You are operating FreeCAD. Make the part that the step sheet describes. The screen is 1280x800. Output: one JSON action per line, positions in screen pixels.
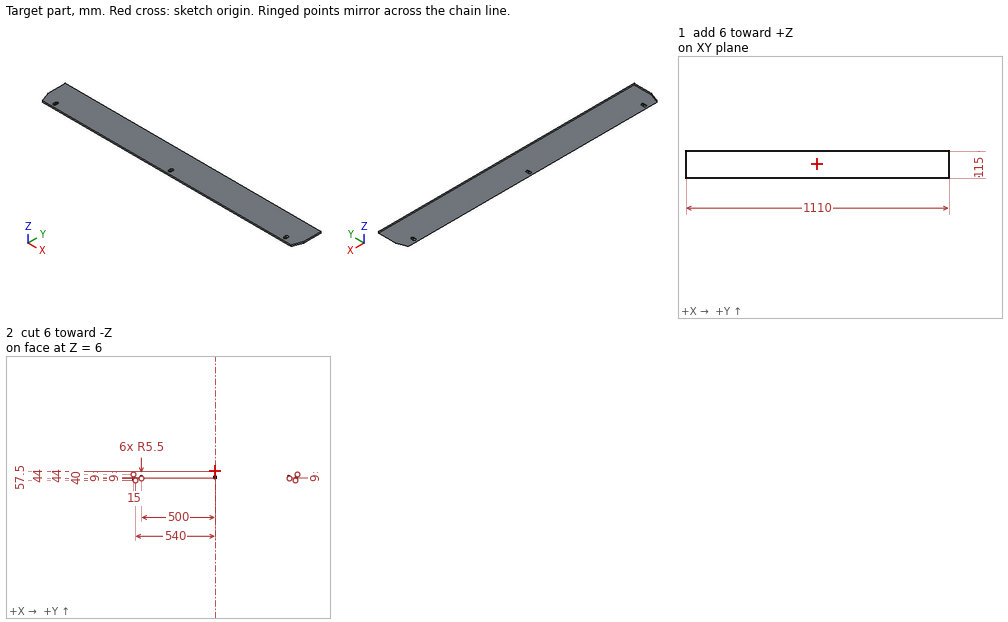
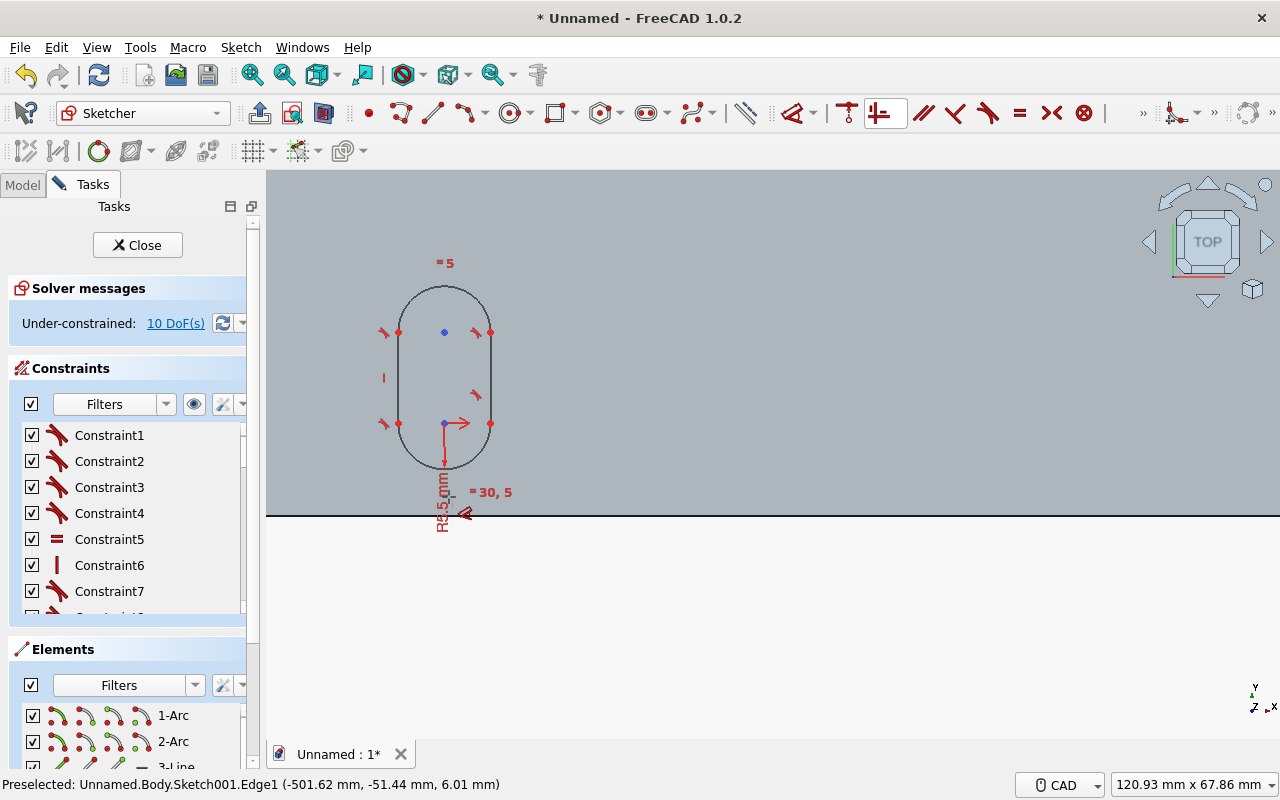
{"action": "left_click", "coordinate": [398, 396]}
{"action": "left_click", "coordinate": [364, 378]}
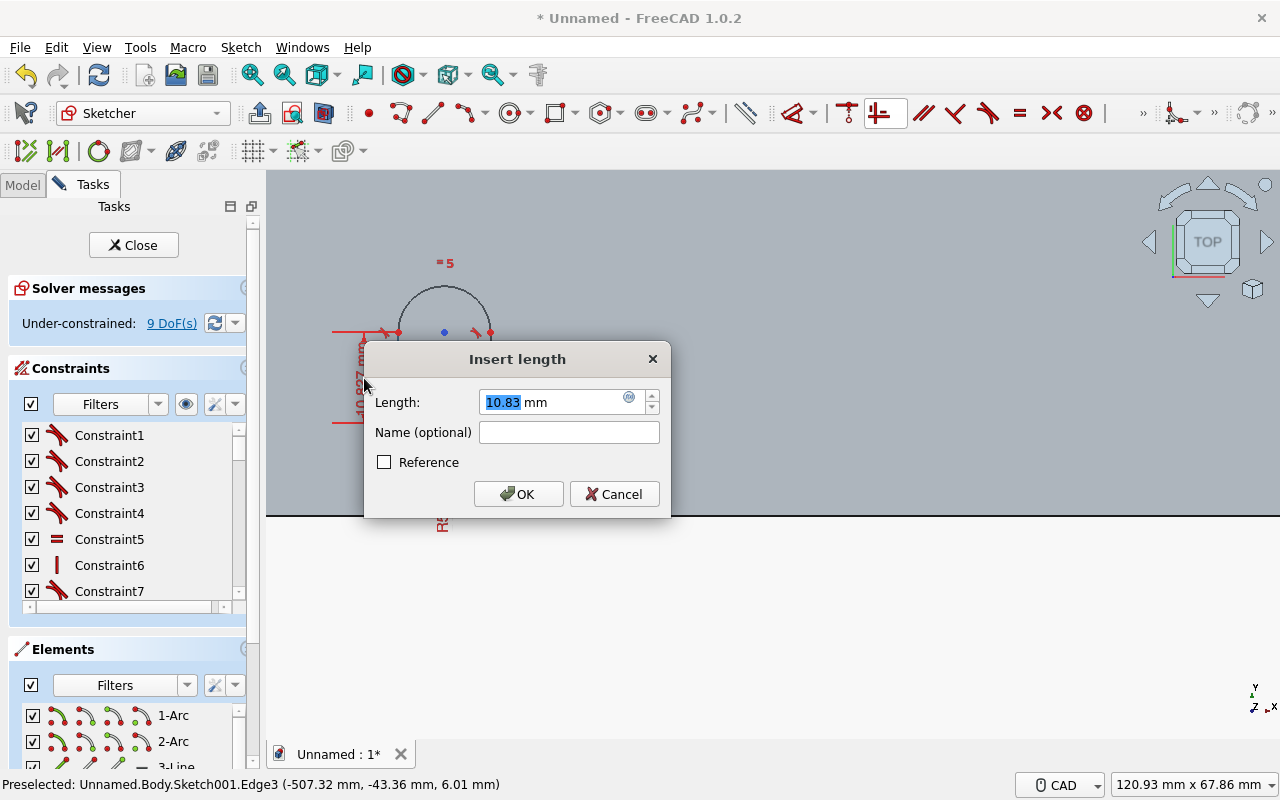
{"action": "type", "text": "9"}
{"action": "key", "text": "Return"}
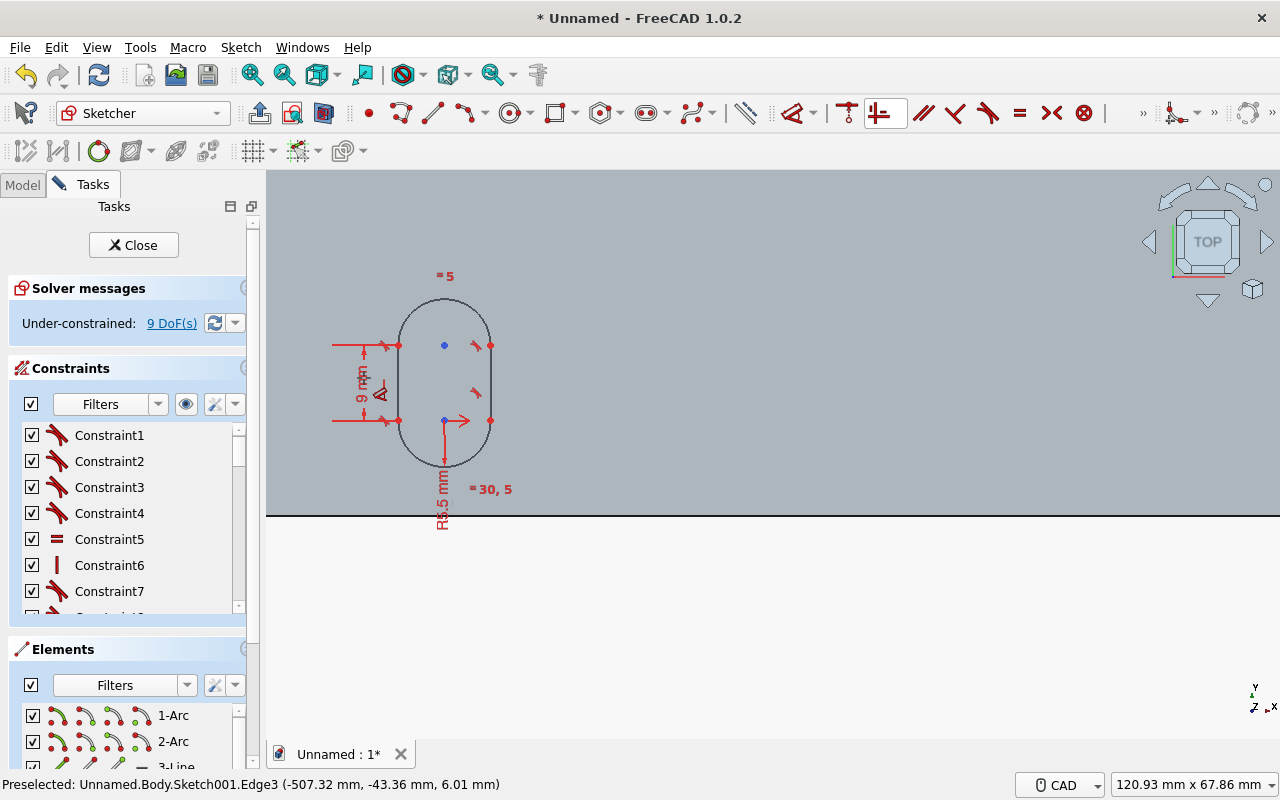
{"action": "scroll", "coordinate": [449, 466], "scroll_direction": "down", "scroll_amount": 14}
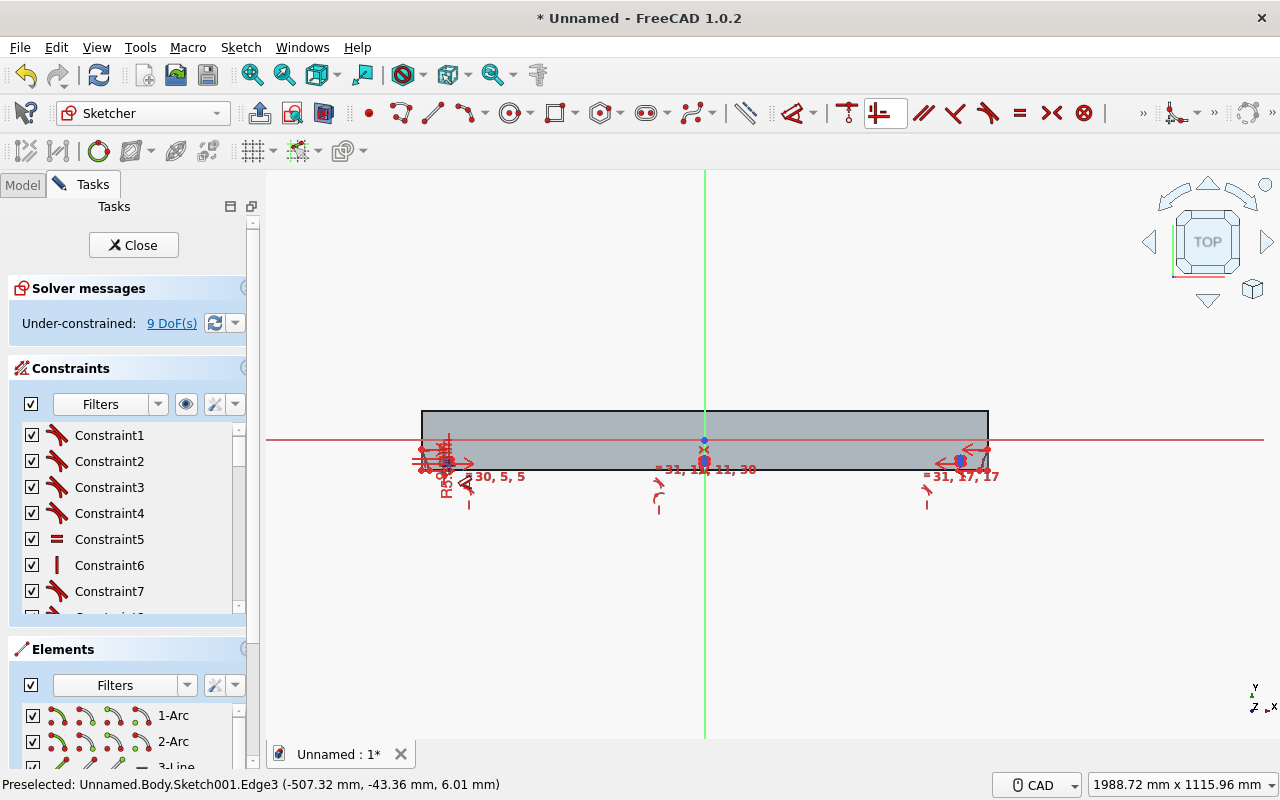
{"action": "scroll", "coordinate": [702, 462], "scroll_direction": "up", "scroll_amount": 13}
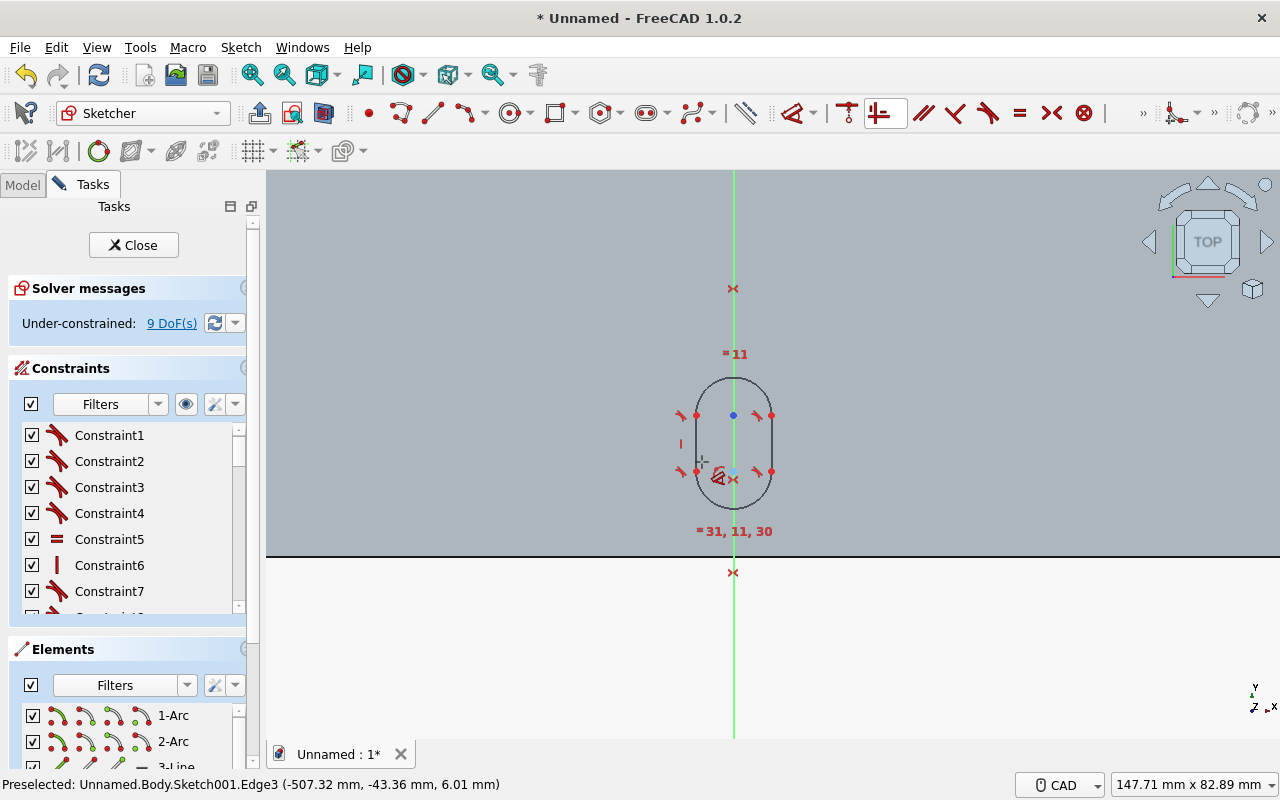
{"action": "left_click", "coordinate": [696, 454]}
{"action": "left_click", "coordinate": [662, 443]}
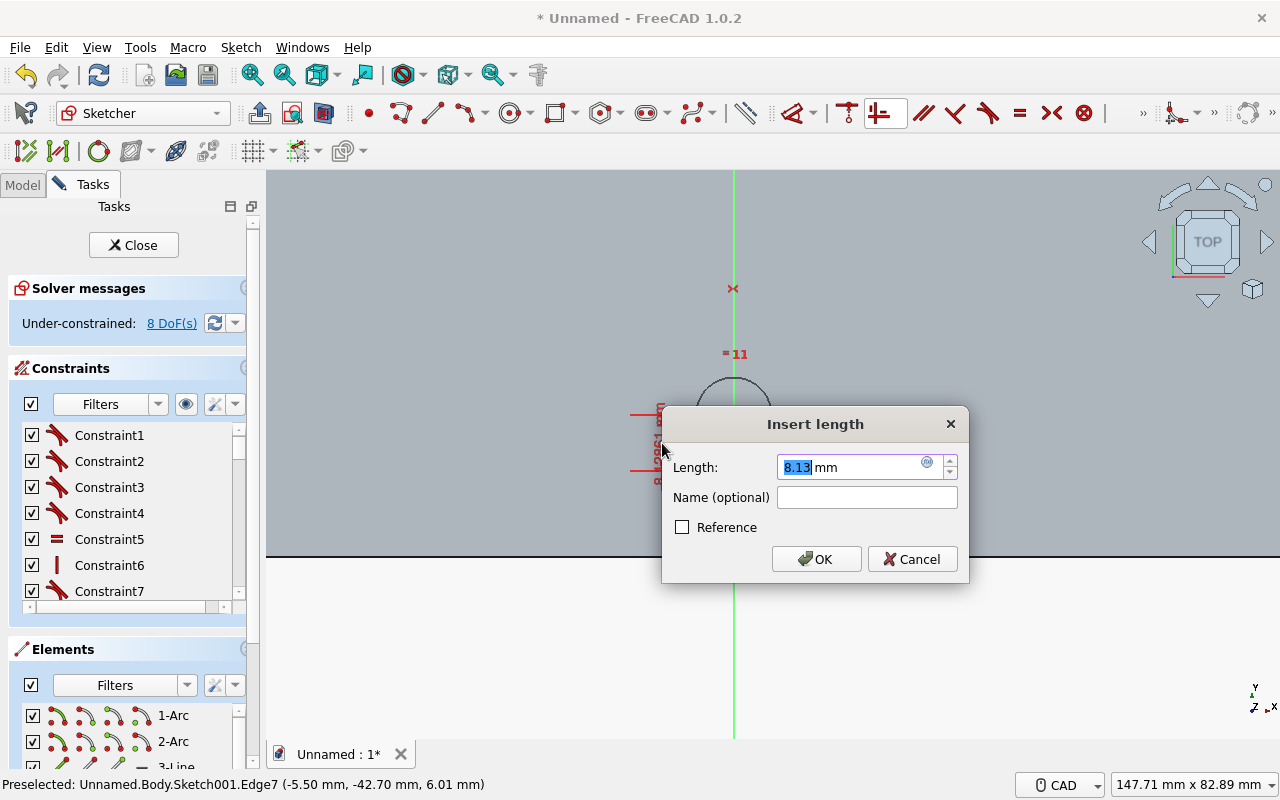
{"action": "type", "text": "9"}
{"action": "key", "text": "Return"}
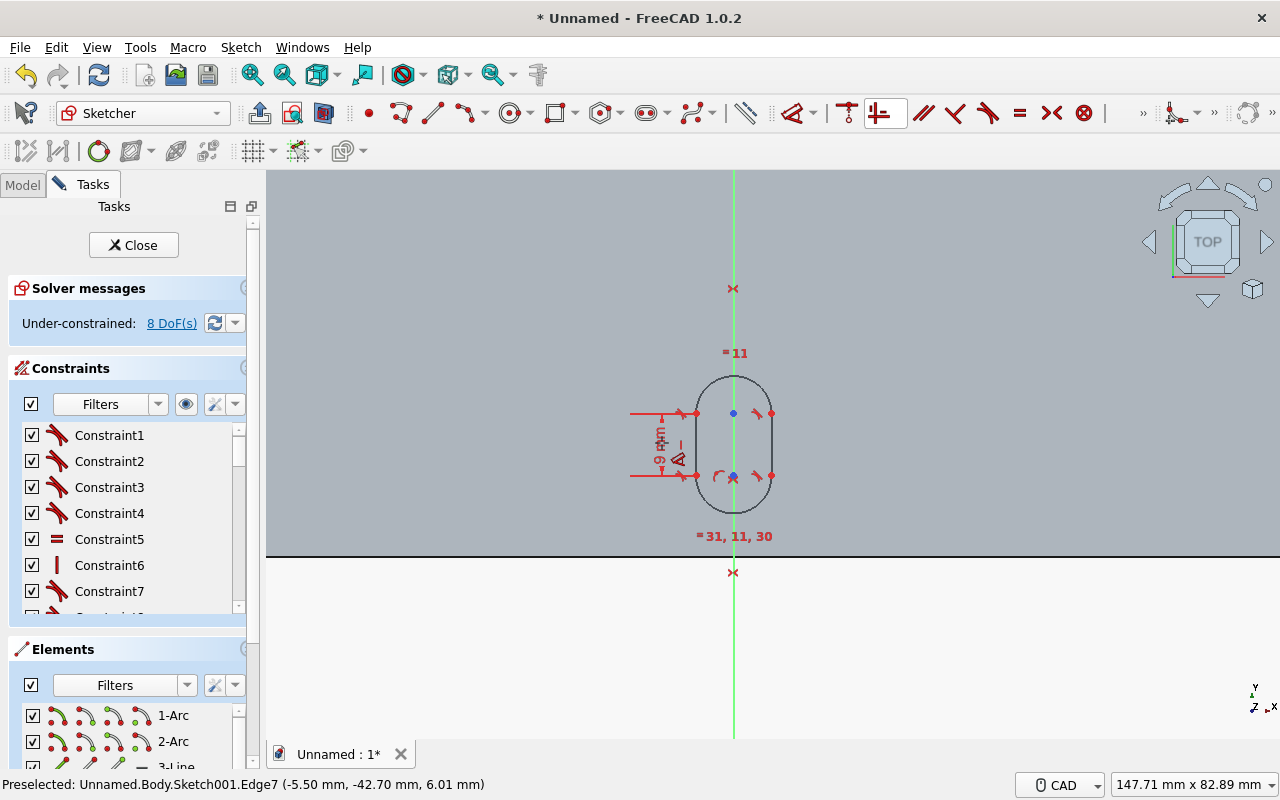
{"action": "scroll", "coordinate": [702, 462], "scroll_direction": "down", "scroll_amount": 13}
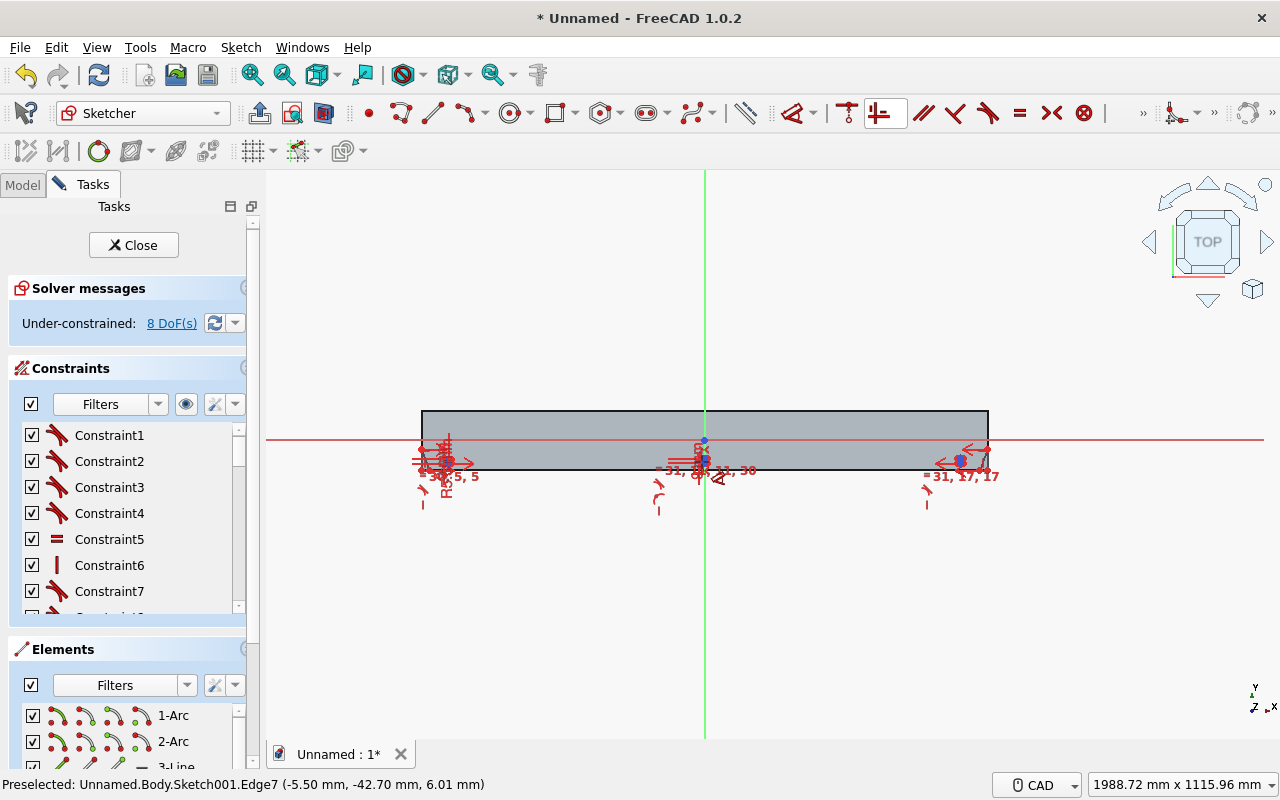
{"action": "scroll", "coordinate": [958, 462], "scroll_direction": "up", "scroll_amount": 11}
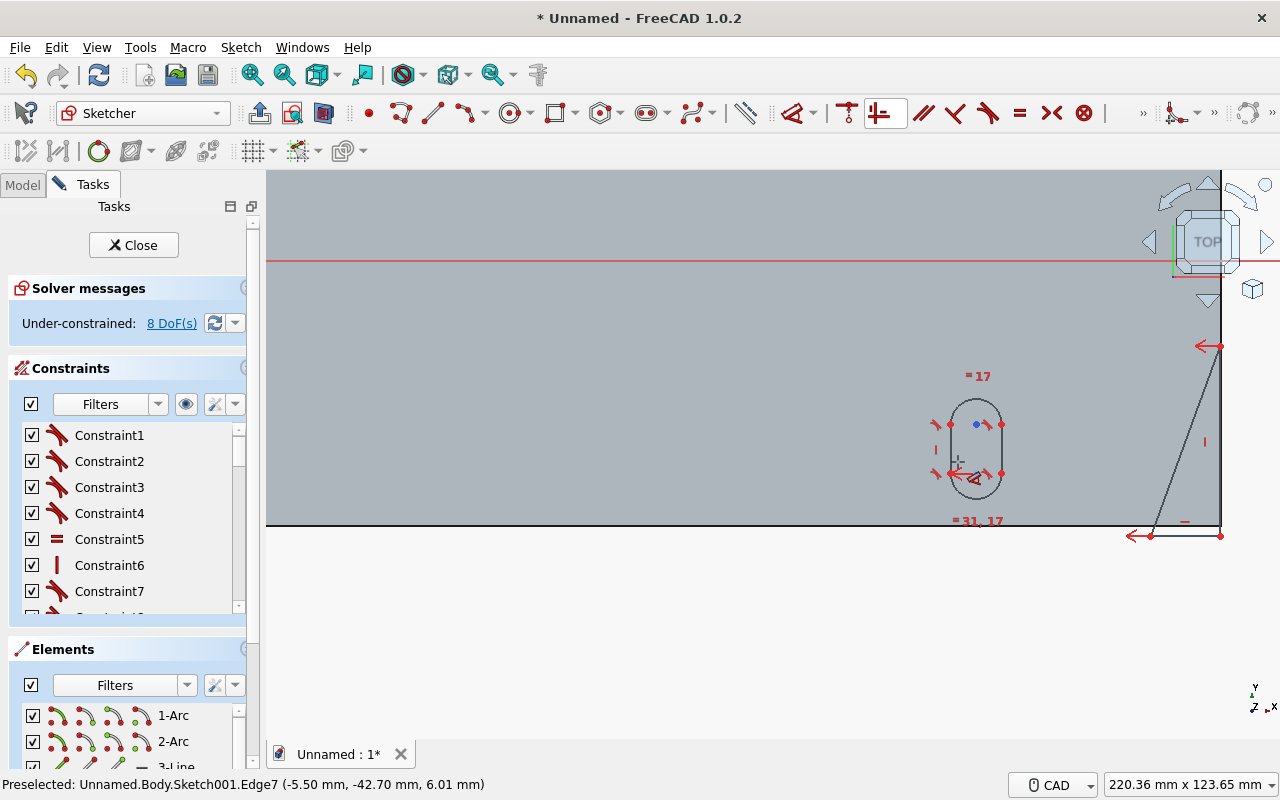
{"action": "left_click", "coordinate": [951, 459]}
{"action": "left_click", "coordinate": [985, 449]}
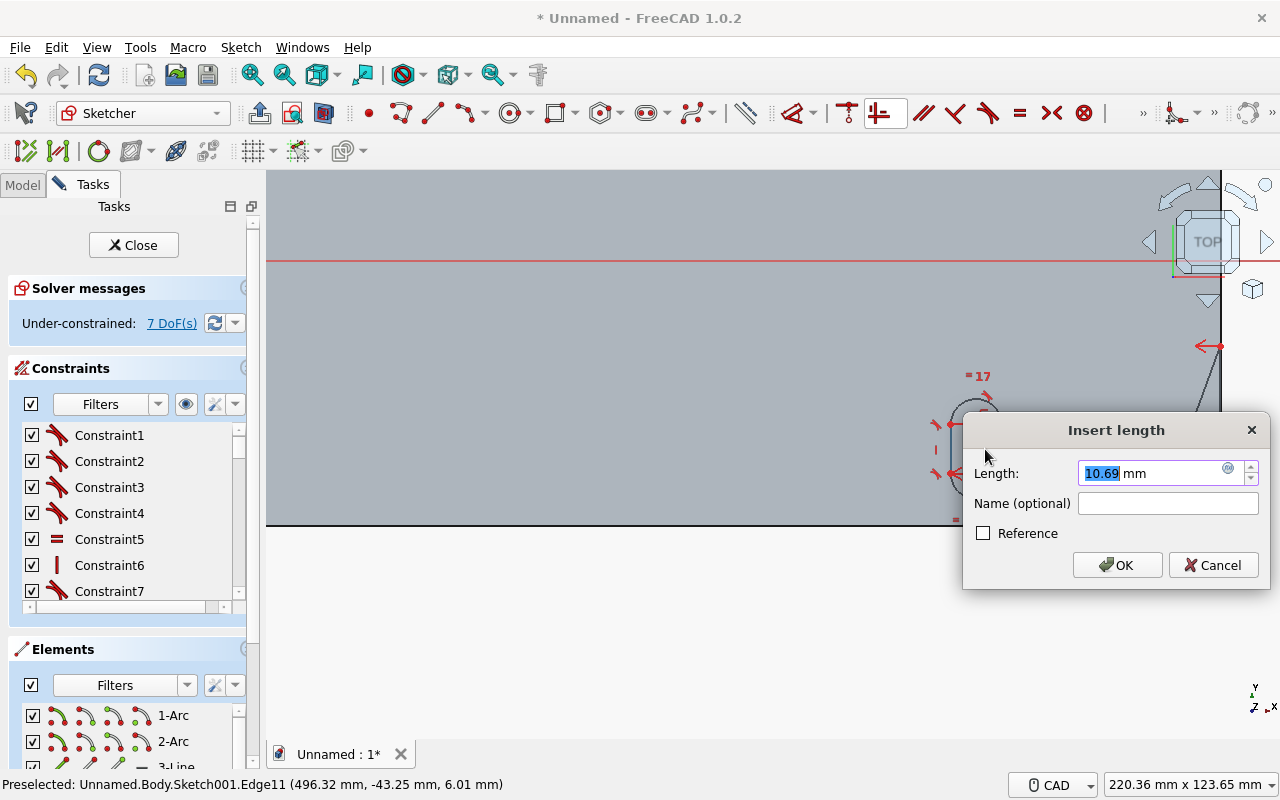
{"action": "type", "text": "9"}
{"action": "key", "text": "Return"}